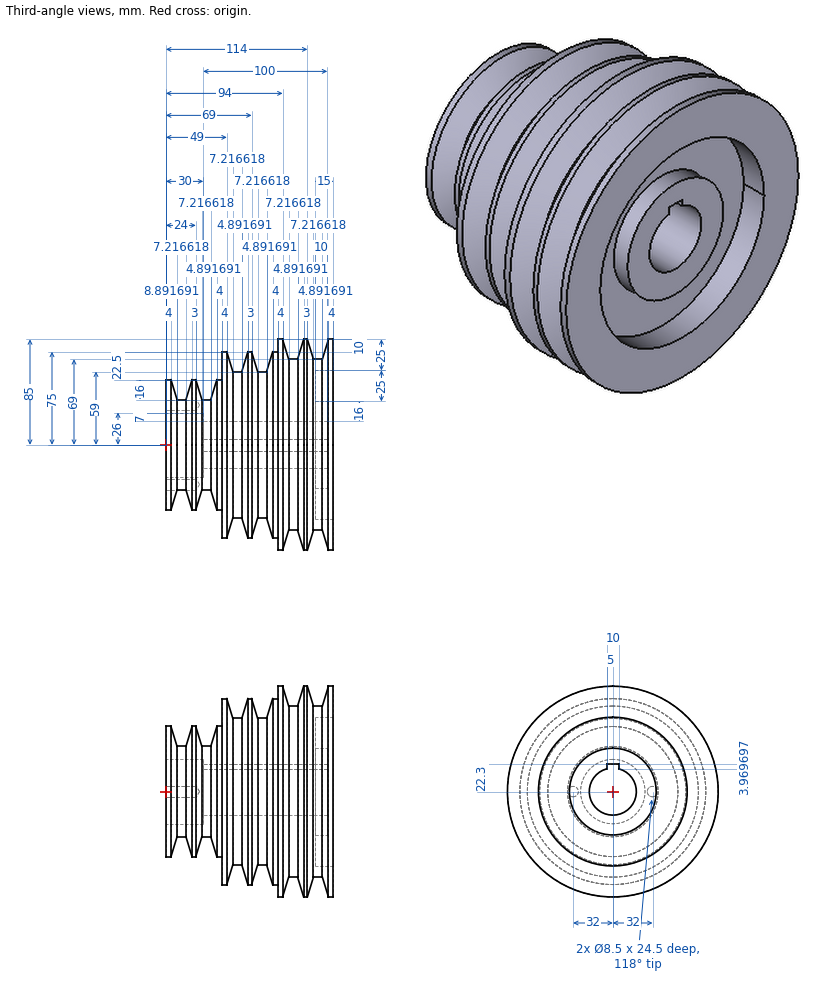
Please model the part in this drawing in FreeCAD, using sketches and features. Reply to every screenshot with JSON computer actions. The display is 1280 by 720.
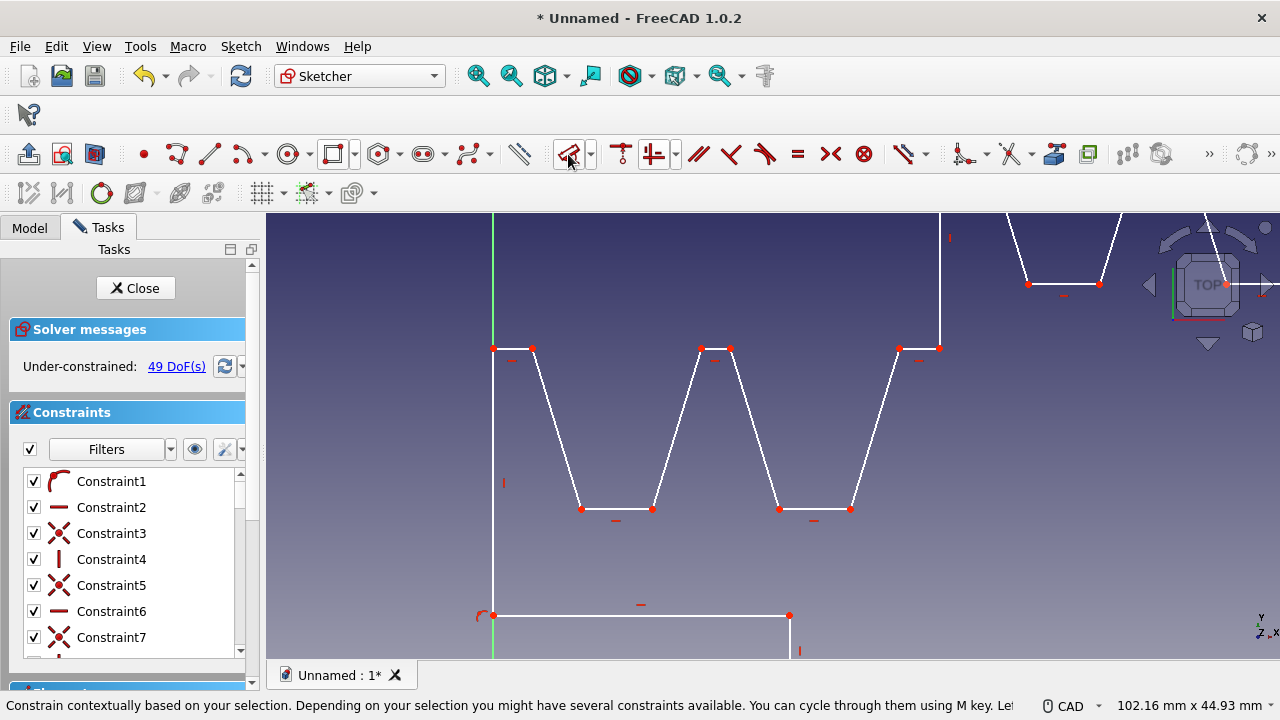
{"action": "left_click", "coordinate": [790, 629]}
{"action": "left_click", "coordinate": [756, 629]}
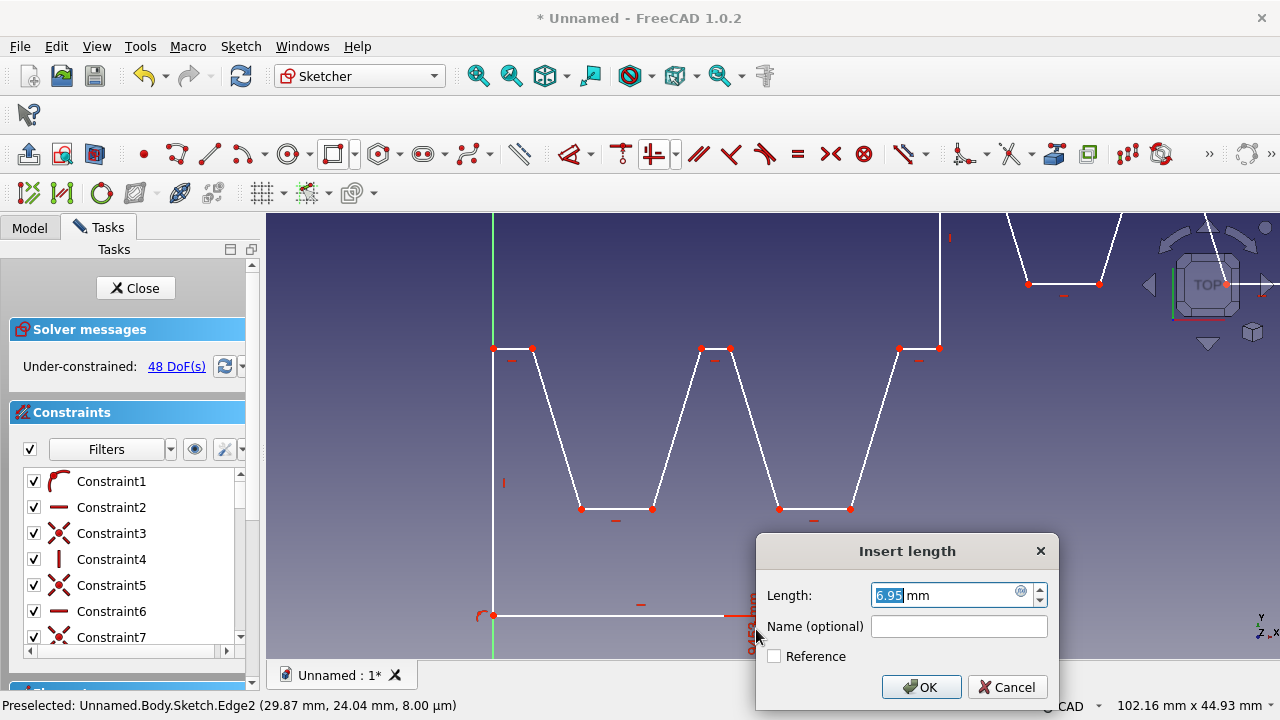
{"action": "type", "text": "7"}
{"action": "key", "text": "Return"}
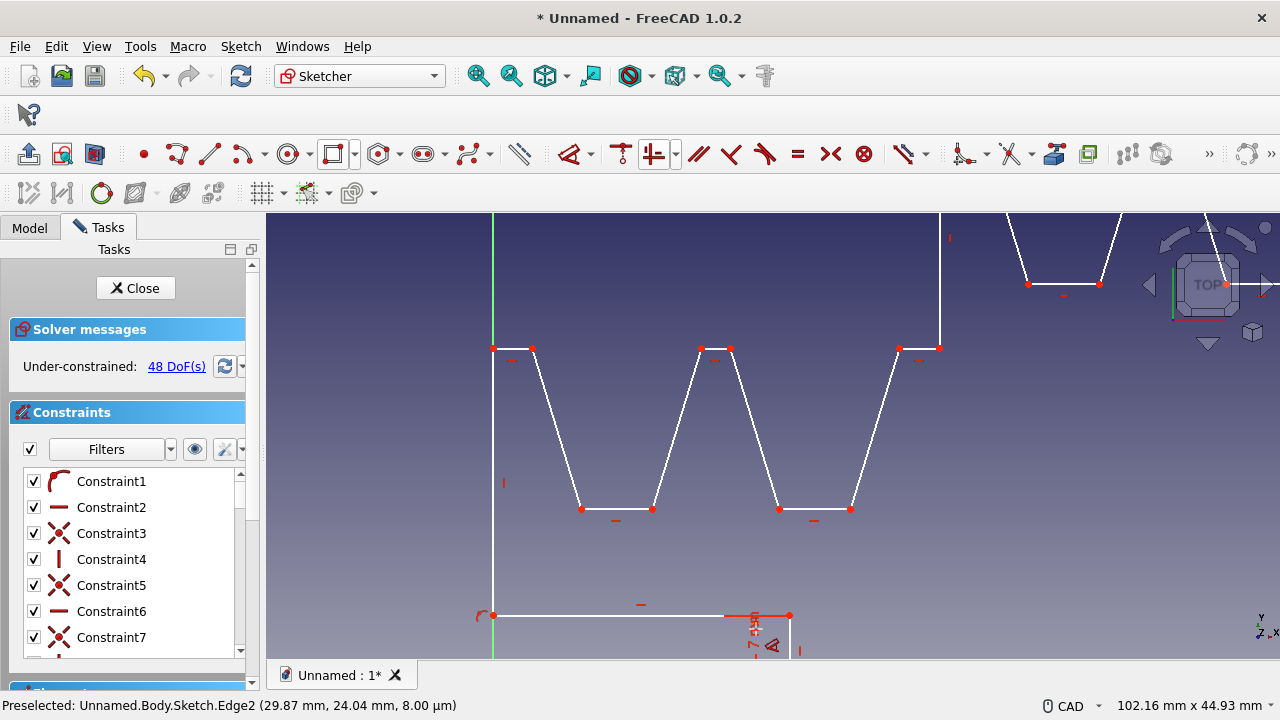
{"action": "scroll", "coordinate": [507, 431], "scroll_direction": "down", "scroll_amount": 6}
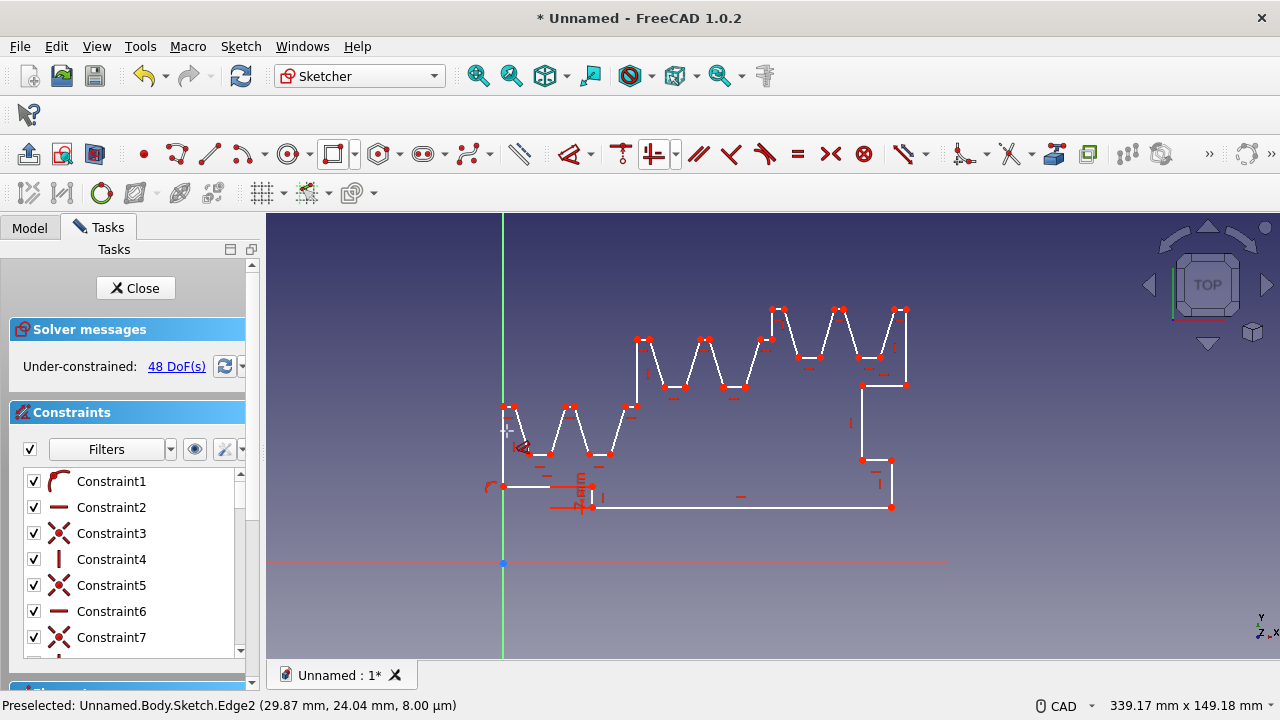
{"action": "scroll", "coordinate": [903, 310], "scroll_direction": "up", "scroll_amount": 8}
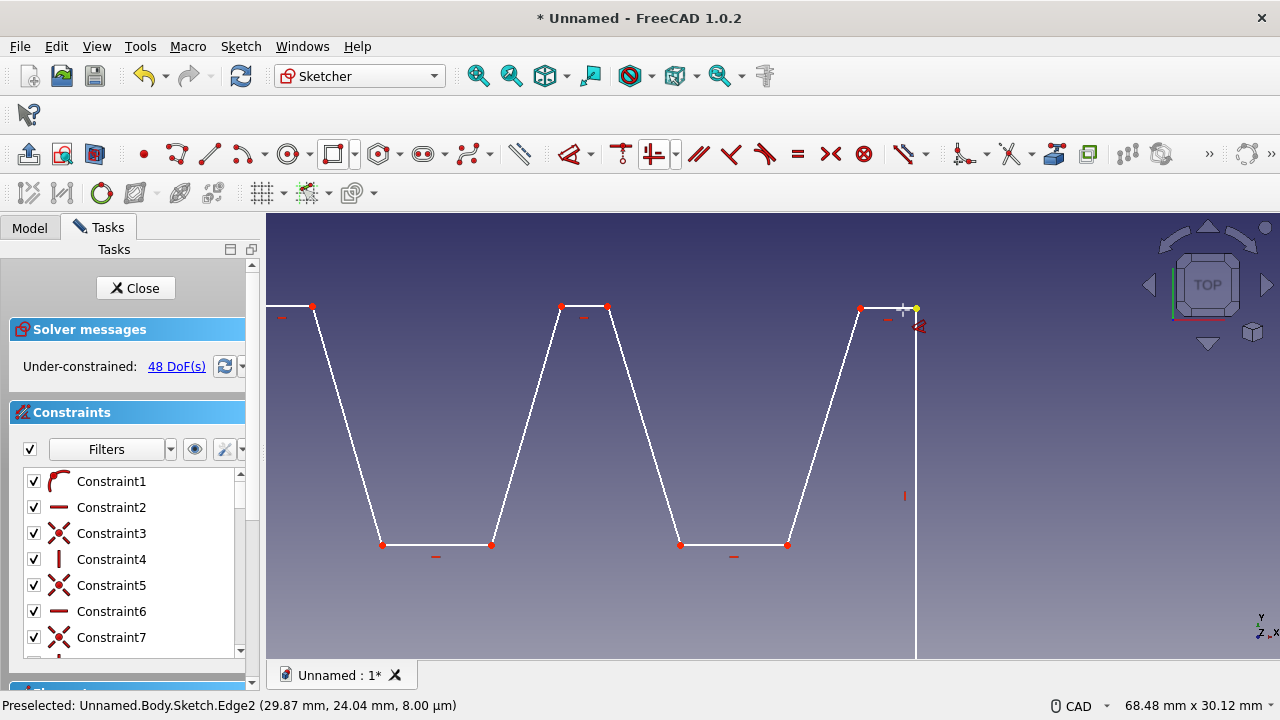
{"action": "left_click", "coordinate": [900, 308]}
{"action": "left_click", "coordinate": [888, 274]}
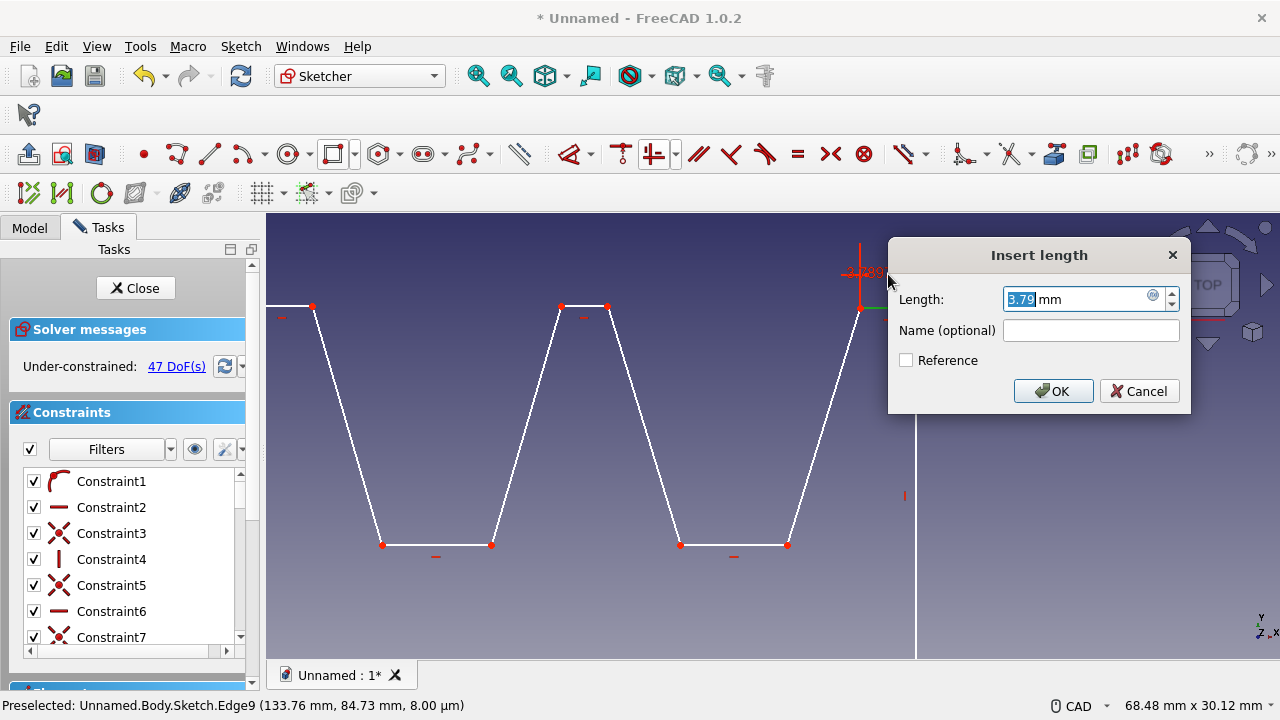
{"action": "type", "text": "4"}
{"action": "key", "text": "Return"}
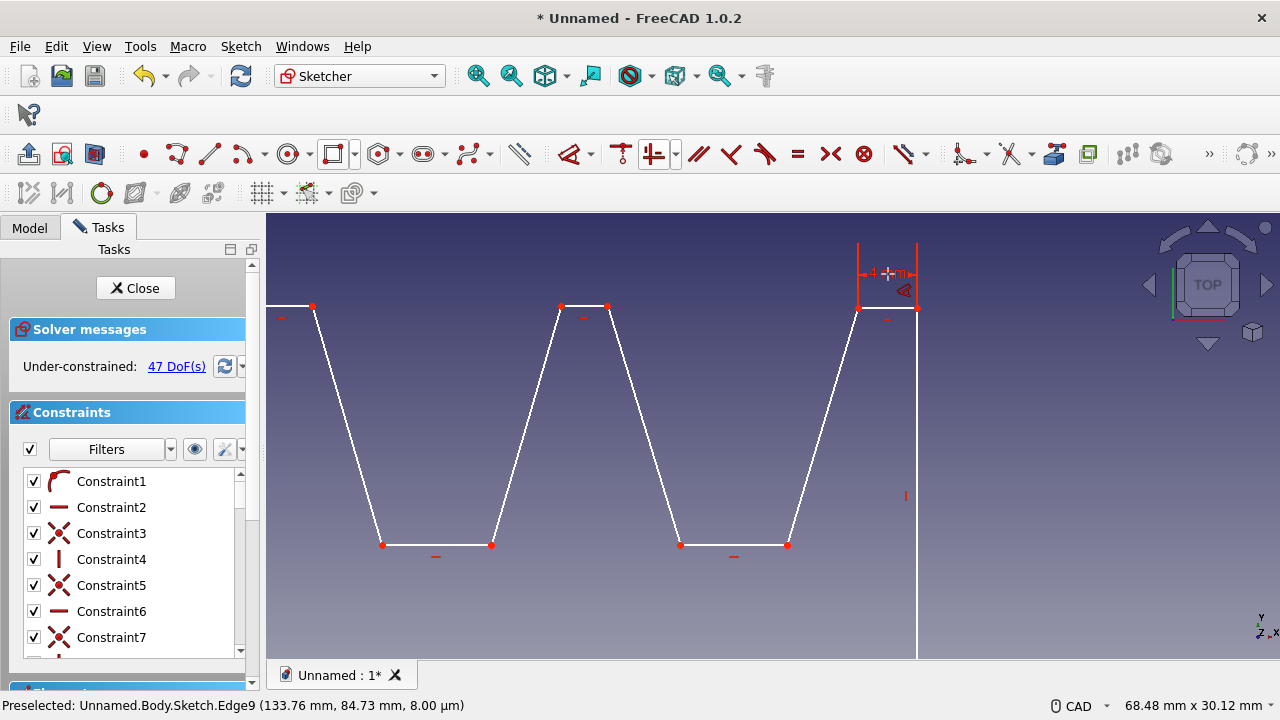
{"action": "left_click", "coordinate": [594, 306]}
{"action": "left_click", "coordinate": [585, 272]}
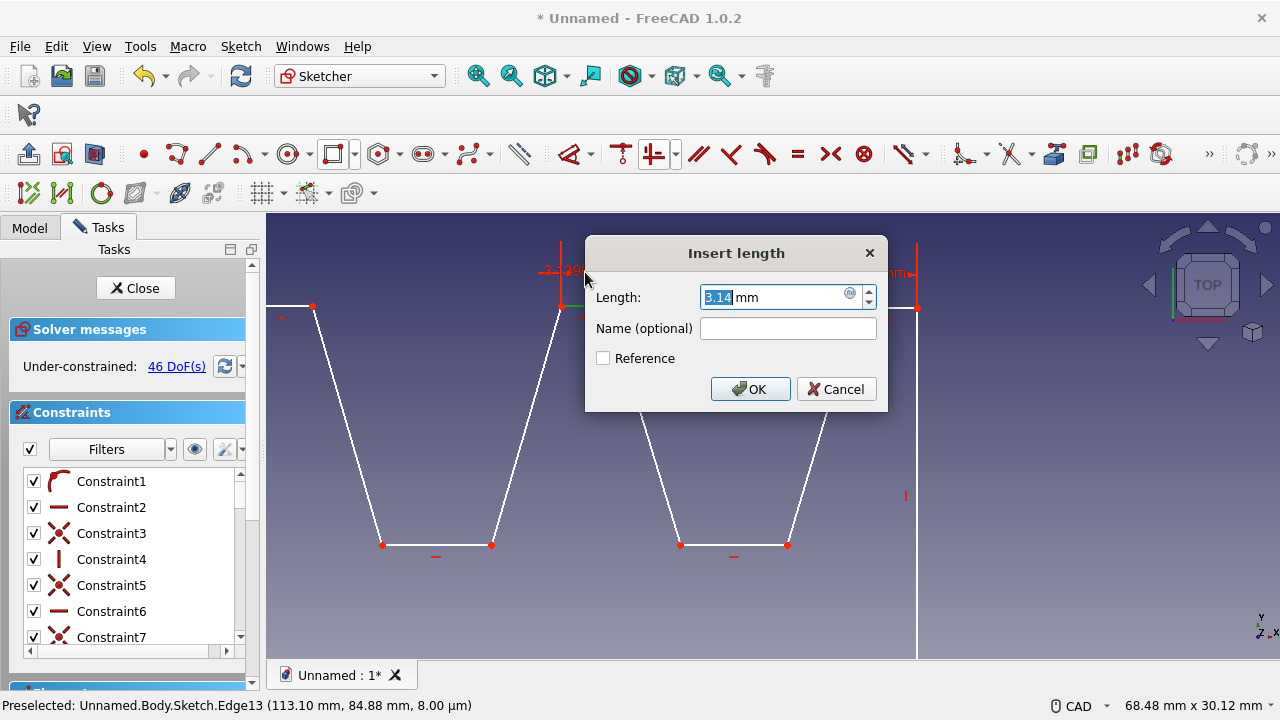
{"action": "type", "text": "3"}
{"action": "key", "text": "Return"}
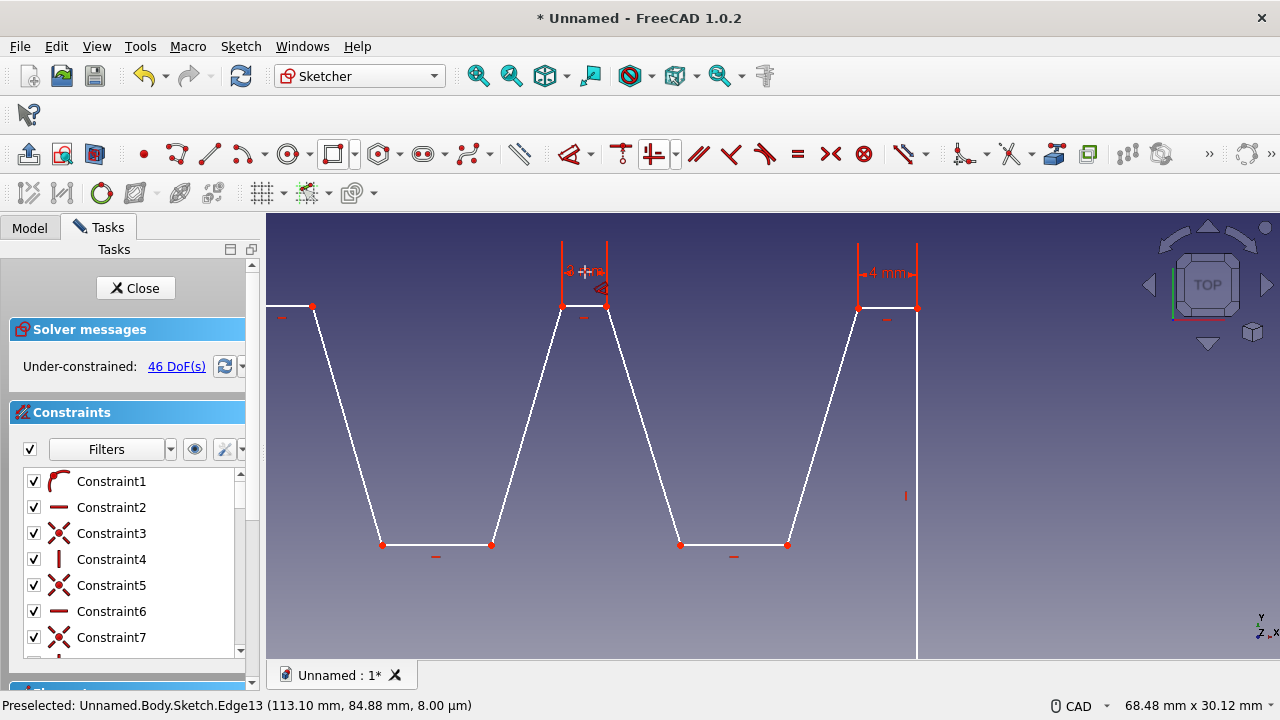
{"action": "left_click", "coordinate": [294, 306]}
{"action": "left_click", "coordinate": [303, 272]}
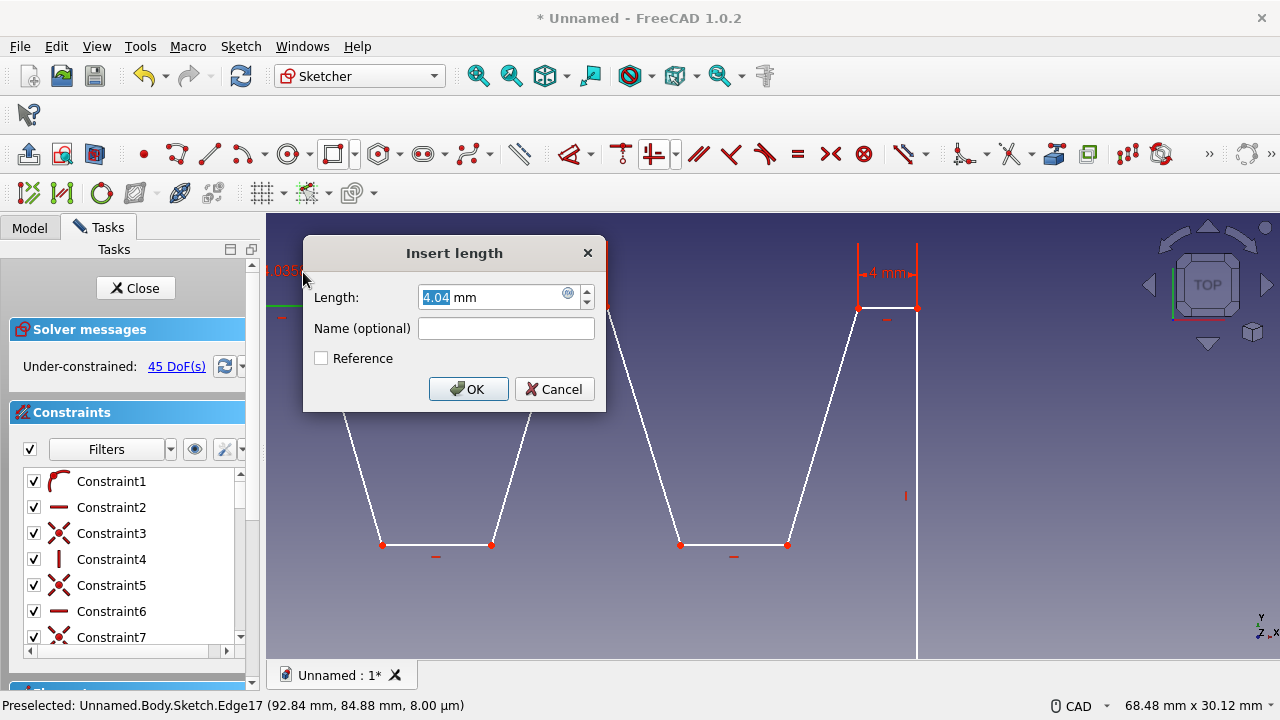
{"action": "type", "text": "4"}
{"action": "key", "text": "Return"}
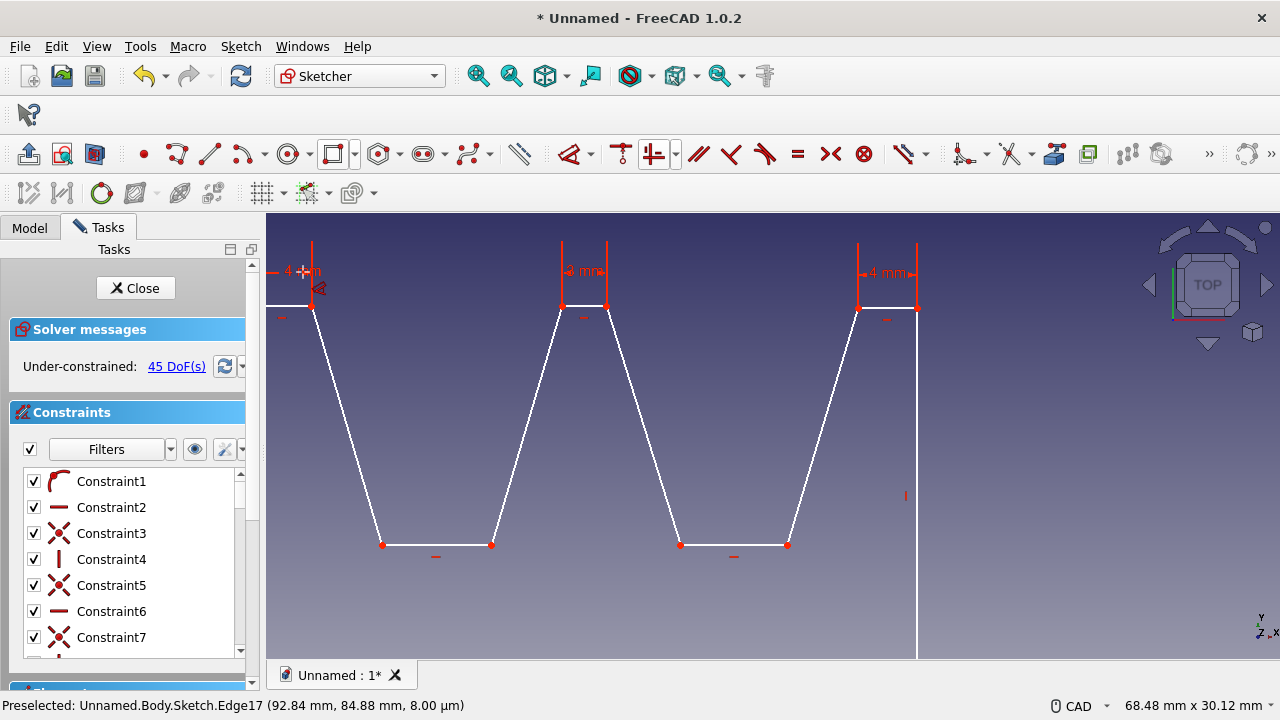
{"action": "scroll", "coordinate": [903, 310], "scroll_direction": "down", "scroll_amount": 8}